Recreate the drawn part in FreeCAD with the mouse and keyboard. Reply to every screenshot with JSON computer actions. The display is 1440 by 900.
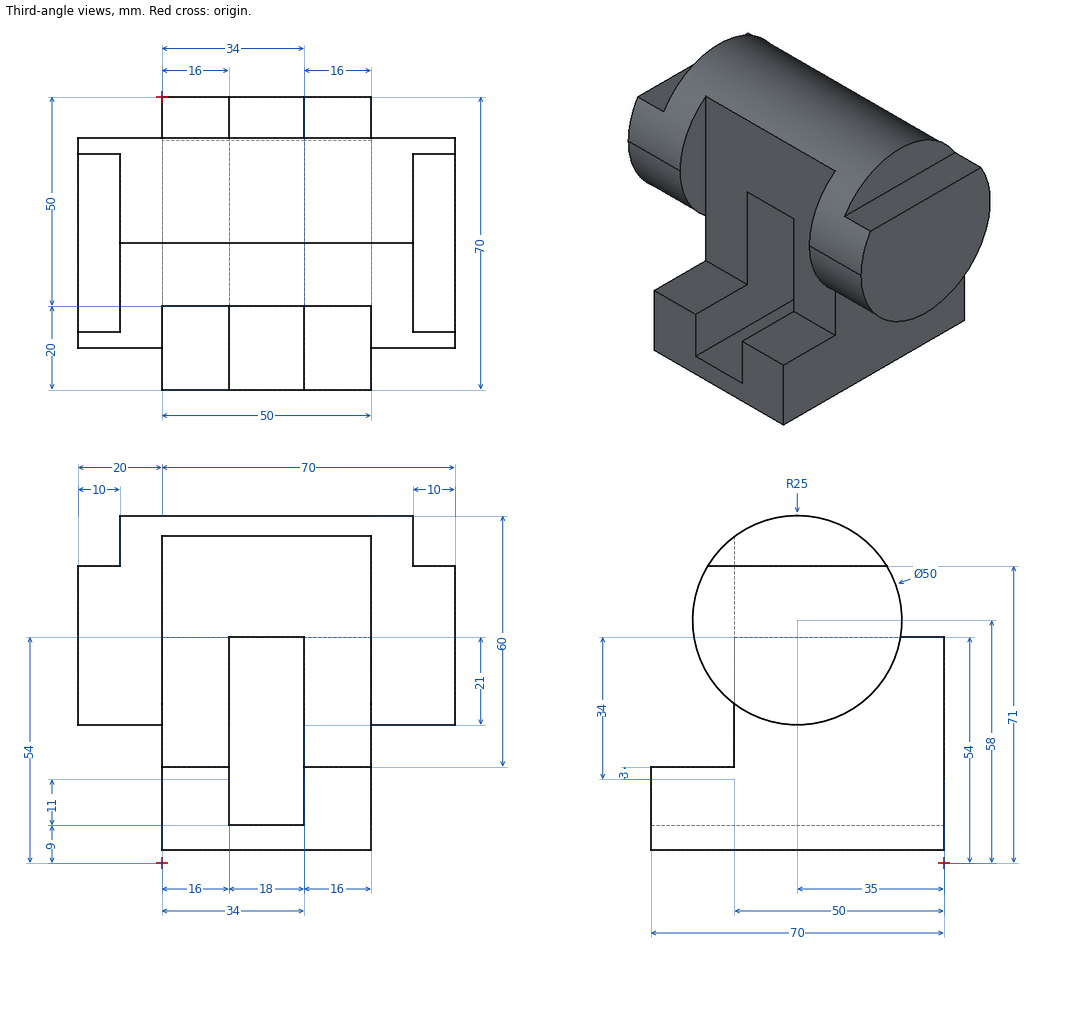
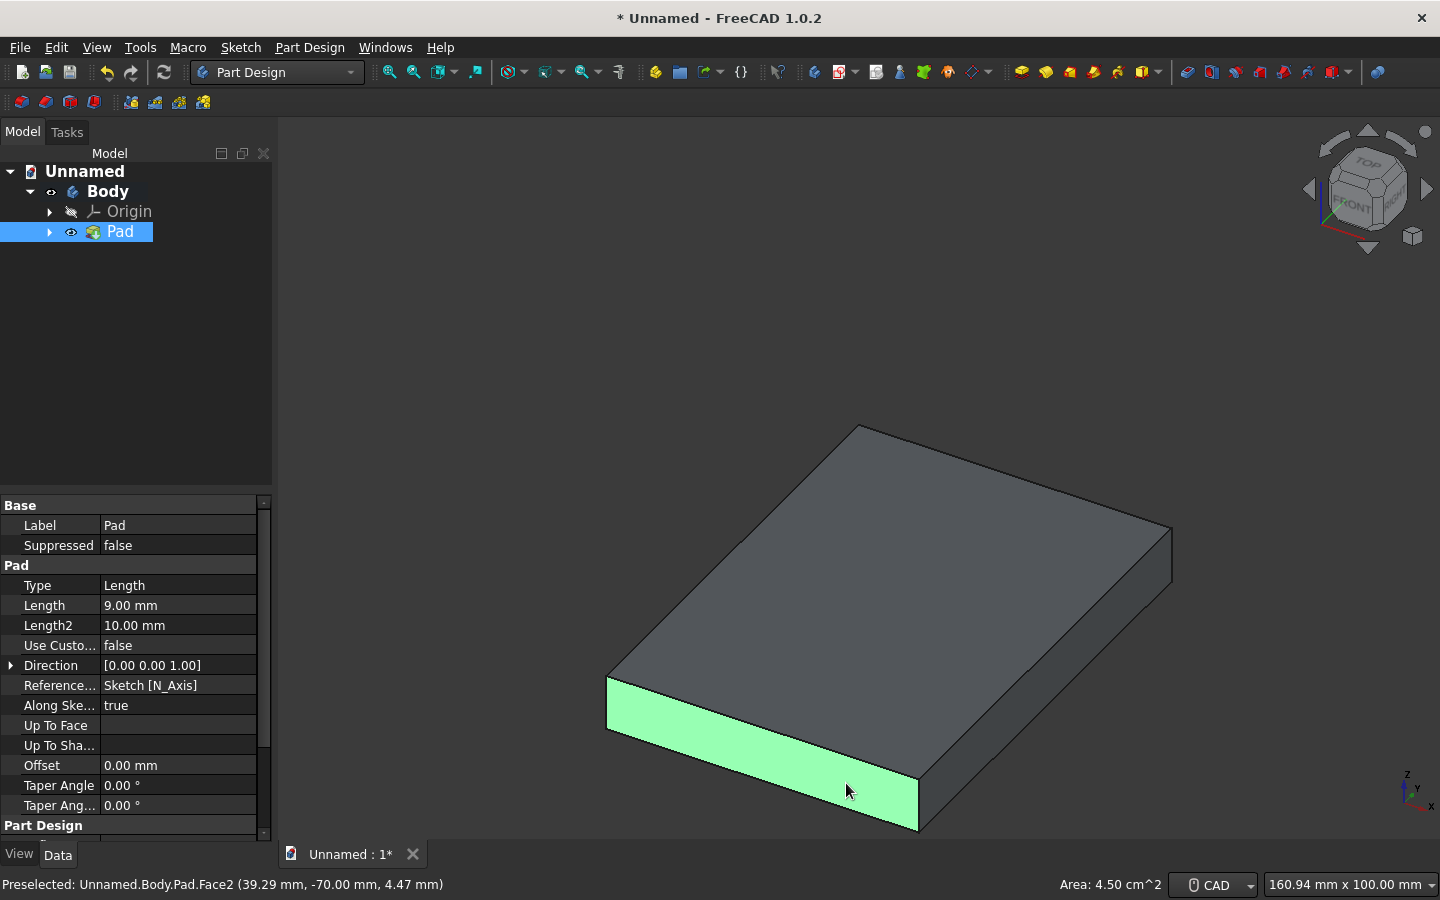
{"action": "left_click", "coordinate": [840, 72]}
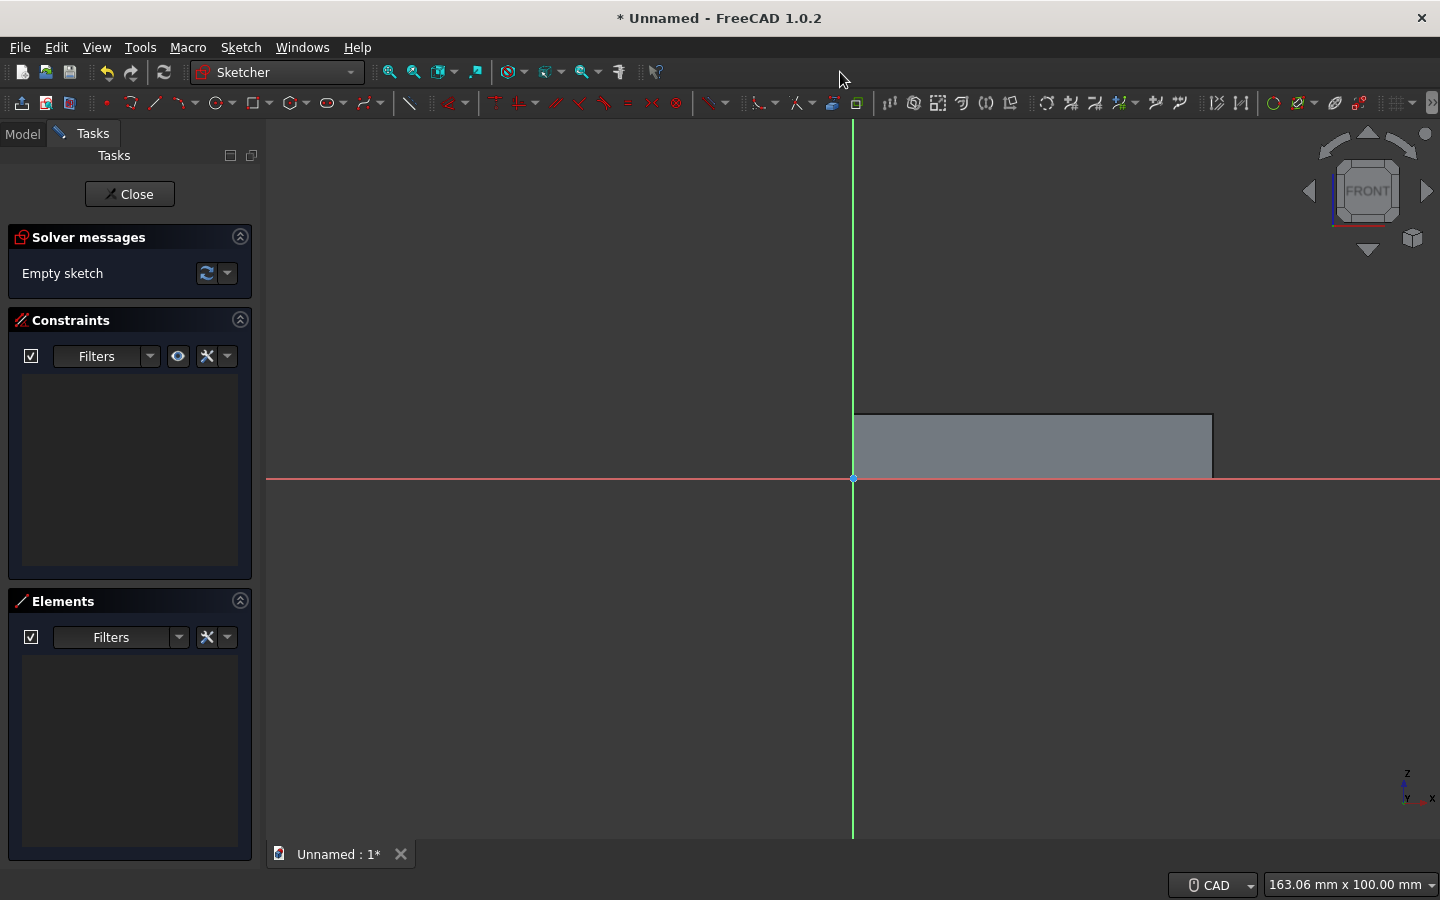
{"action": "scroll", "coordinate": [1275, 319], "scroll_direction": "up", "scroll_amount": 3}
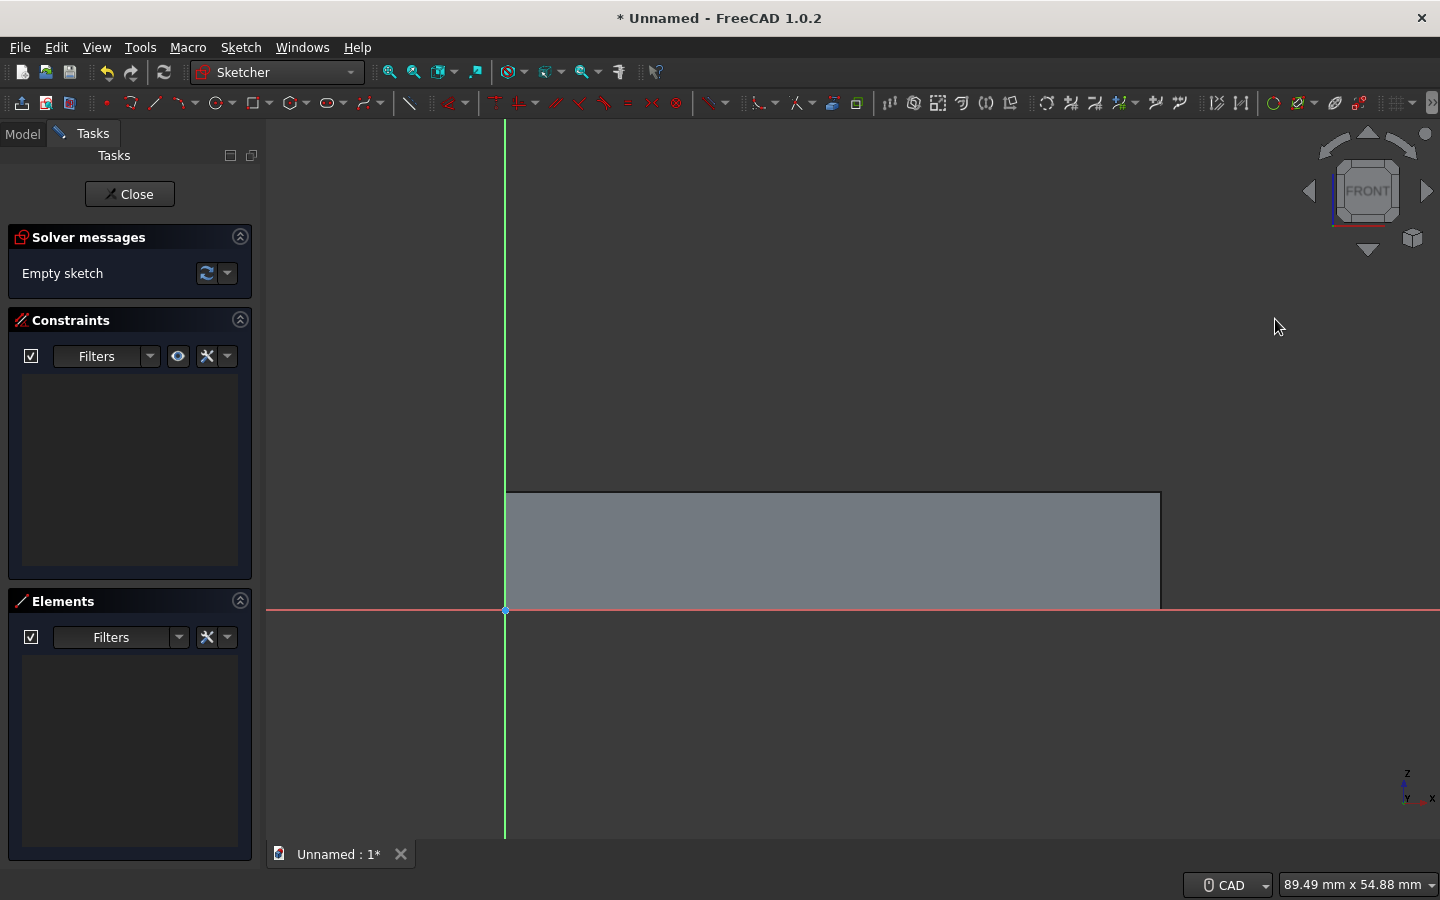
{"action": "key", "text": "g r"}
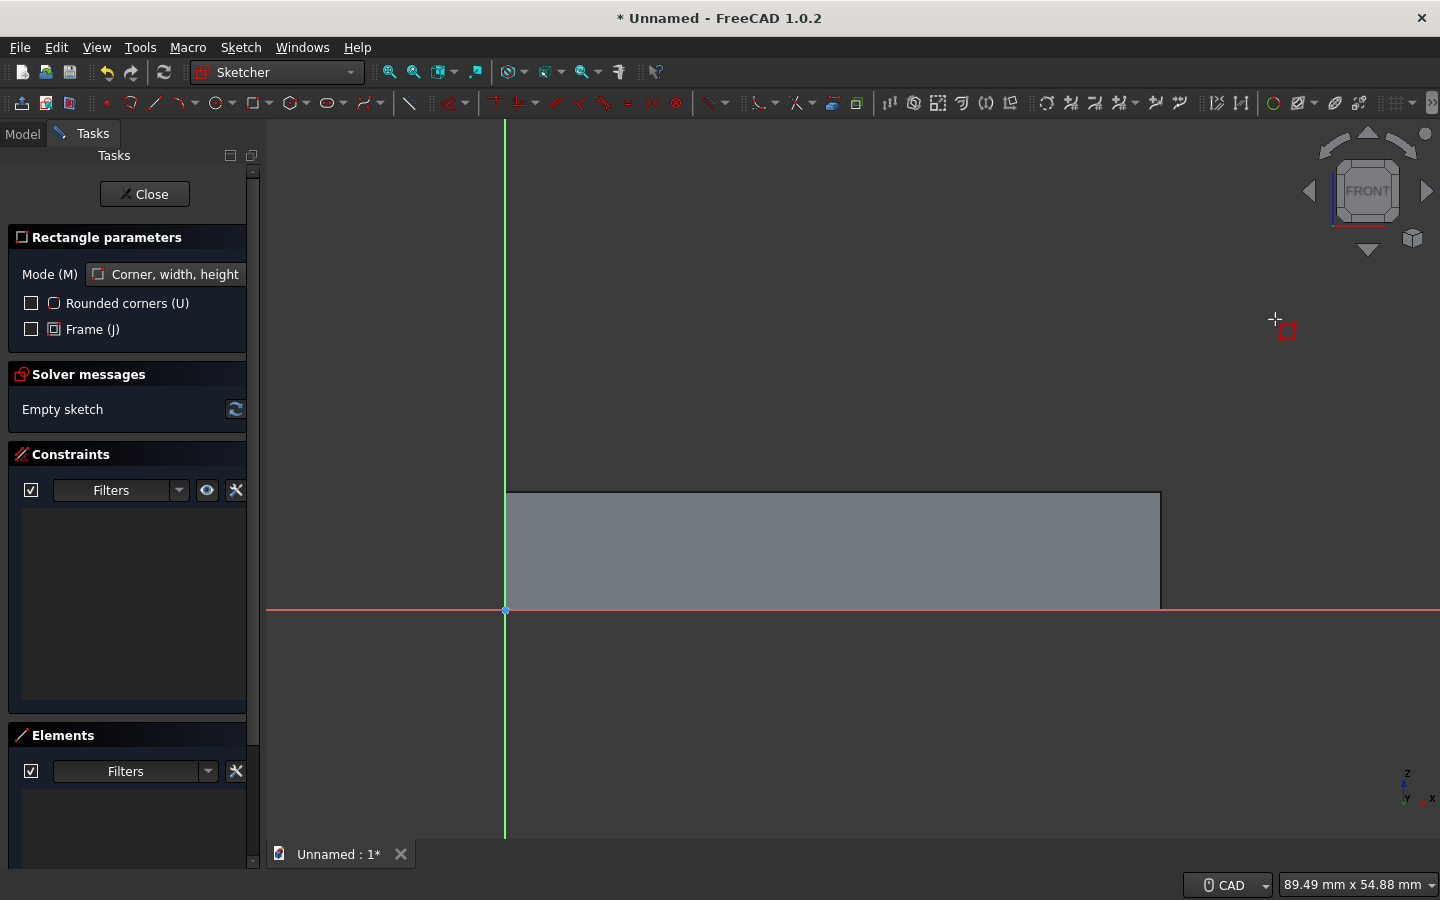
{"action": "left_click", "coordinate": [505, 348]}
{"action": "mouse_move", "coordinate": [715, 492]}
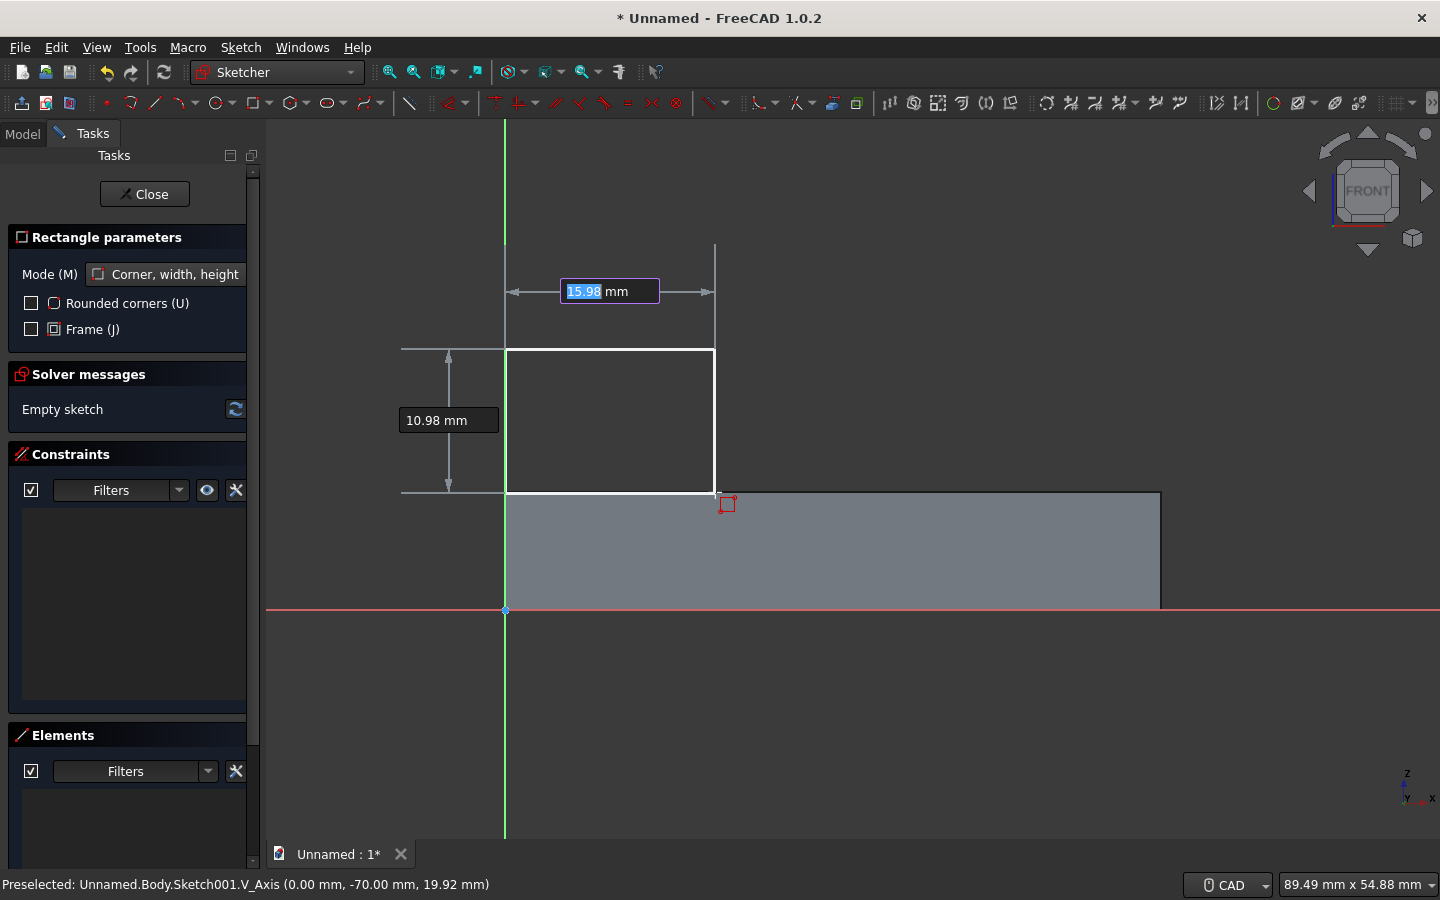
{"action": "type", "text": "16"}
{"action": "key", "text": "Tab"}
{"action": "type", "text": "11"}
{"action": "key", "text": "Return"}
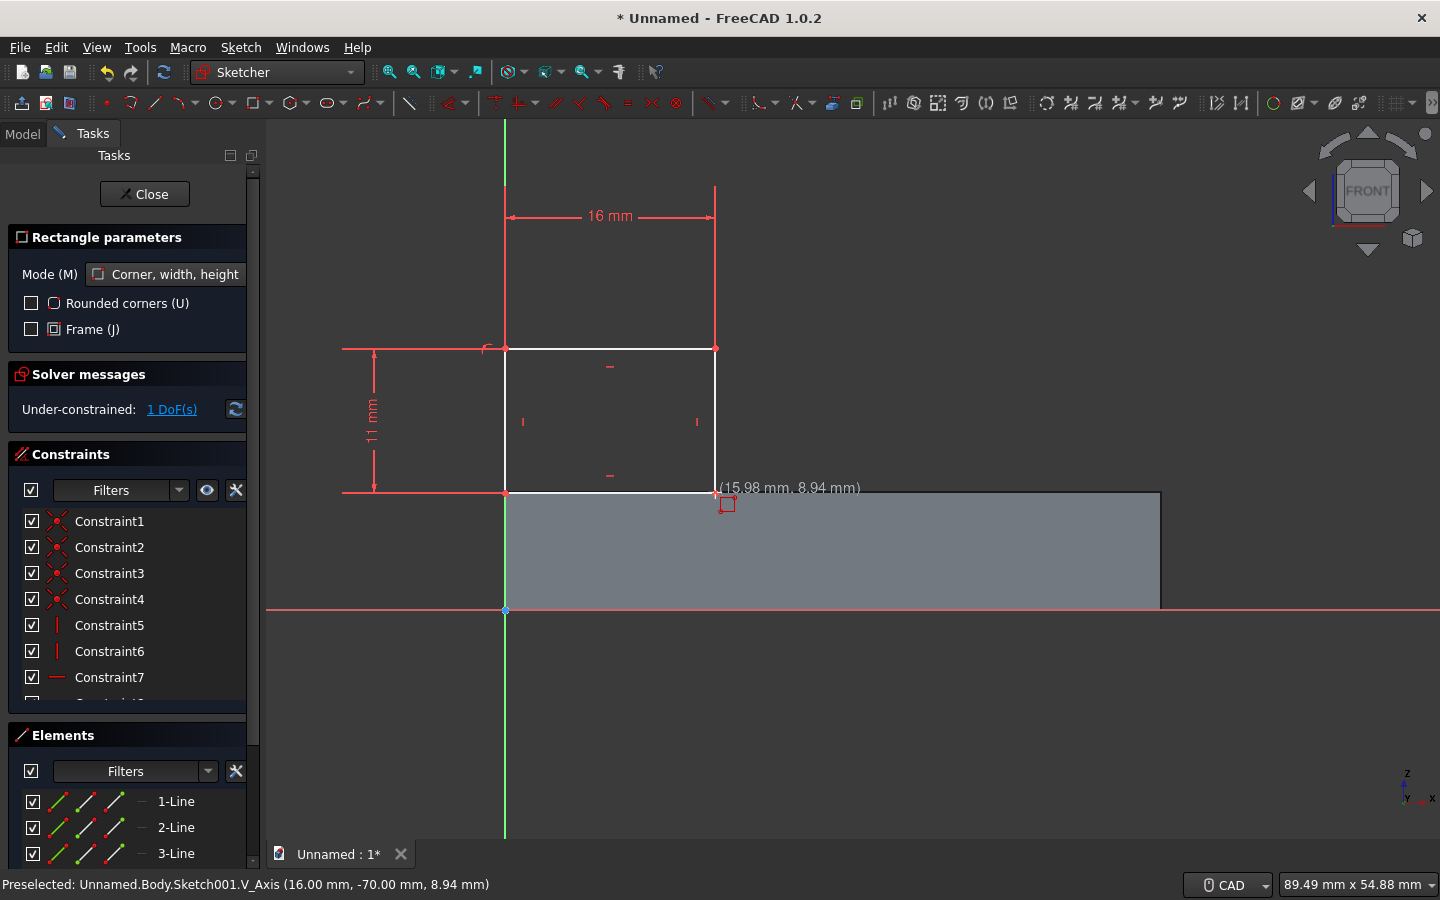
{"action": "left_click", "coordinate": [951, 348]}
{"action": "mouse_move", "coordinate": [1161, 492]}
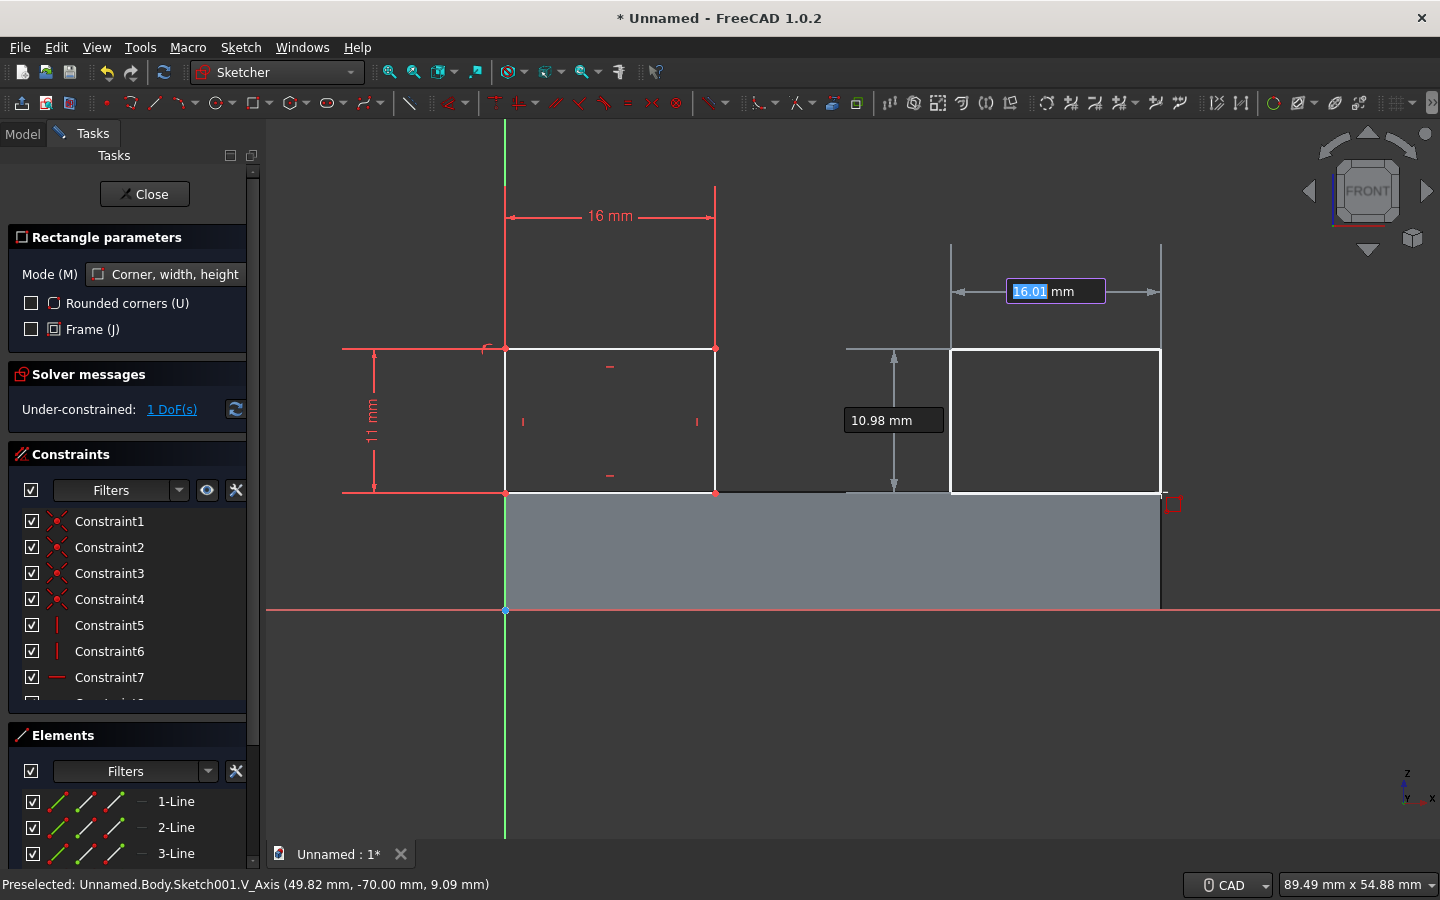
{"action": "type", "text": "16"}
{"action": "key", "text": "Tab"}
{"action": "type", "text": "11"}
{"action": "key", "text": "Return"}
{"action": "key", "text": "Escape"}